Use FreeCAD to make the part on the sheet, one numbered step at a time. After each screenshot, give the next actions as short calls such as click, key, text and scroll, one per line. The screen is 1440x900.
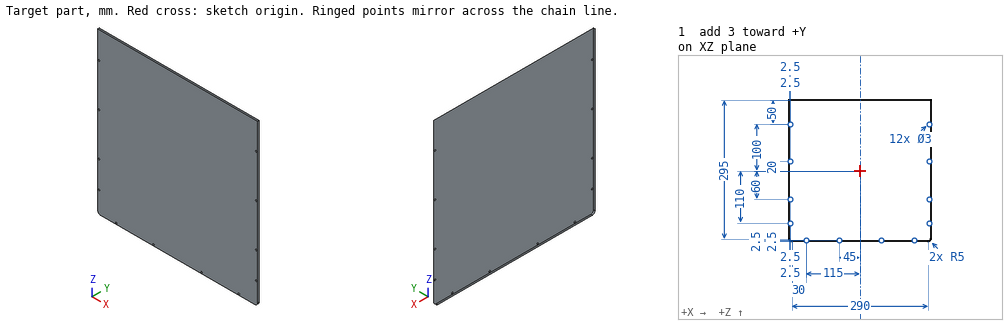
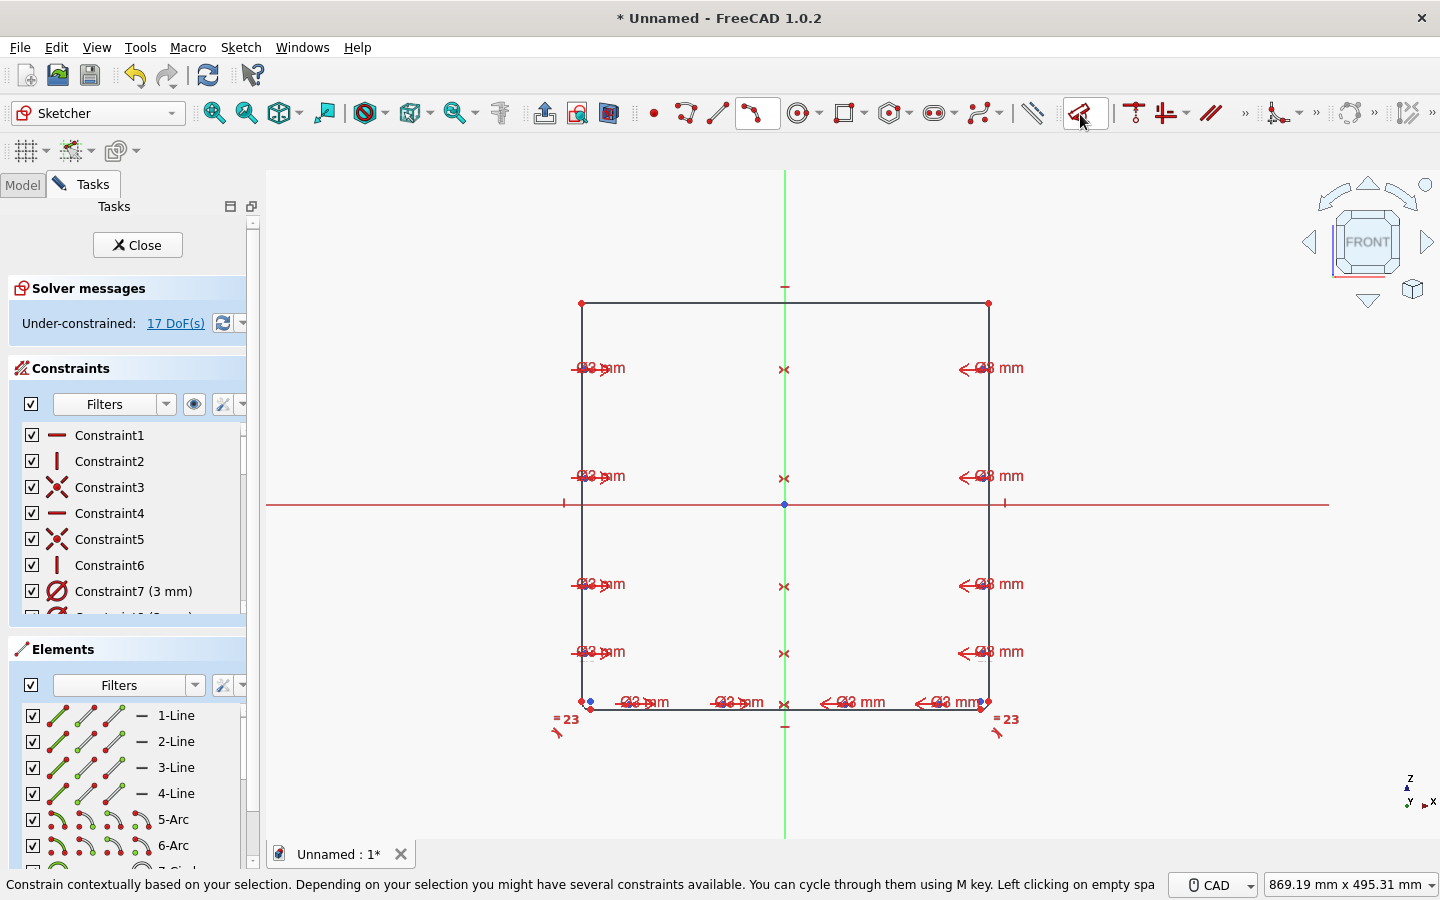
scroll(584, 708, up, 9)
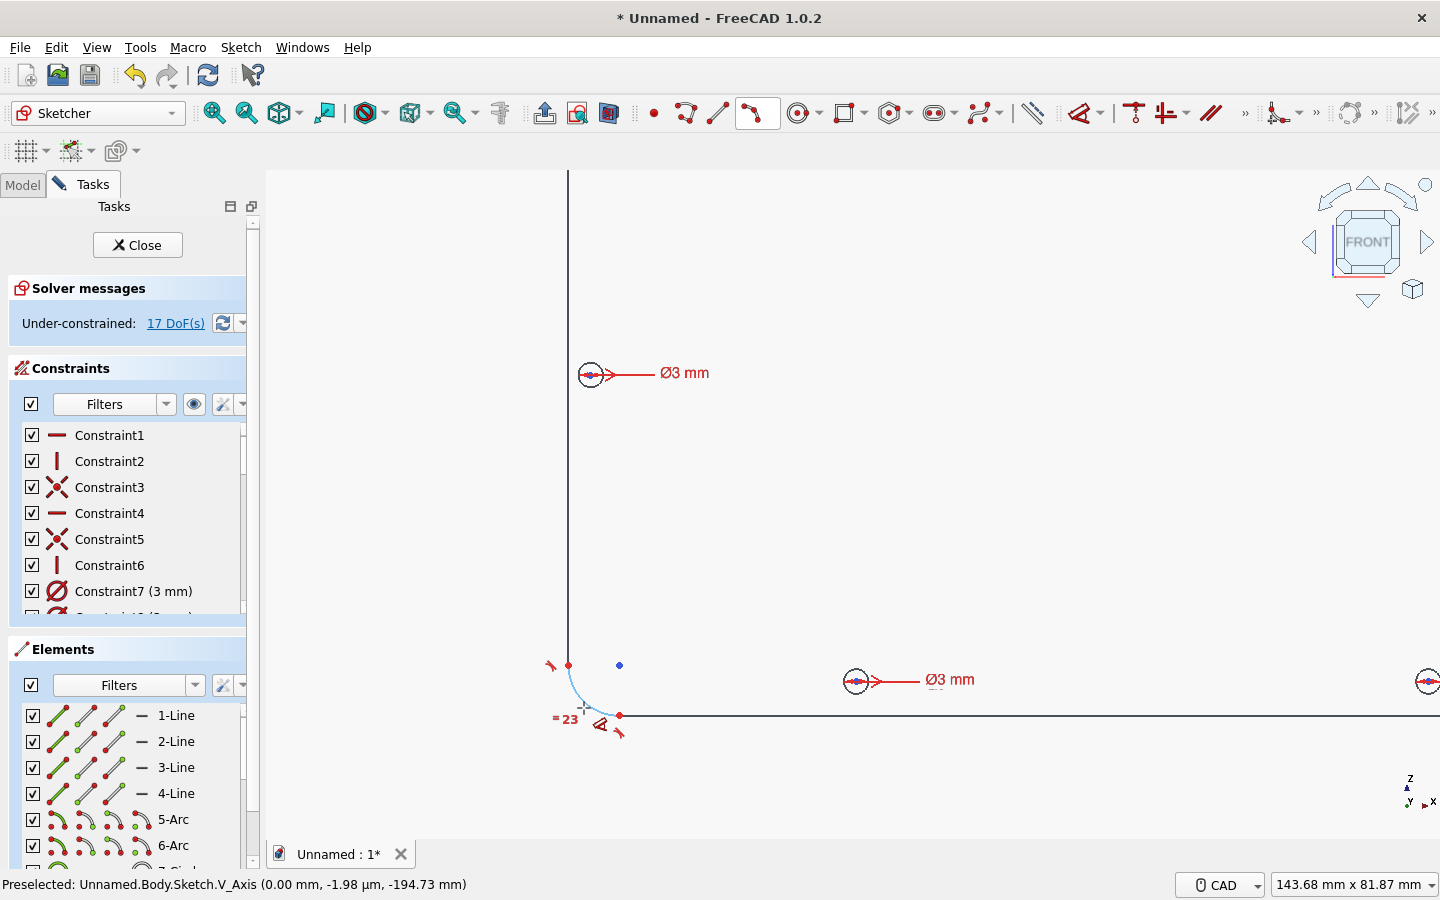
click(583, 701)
click(560, 724)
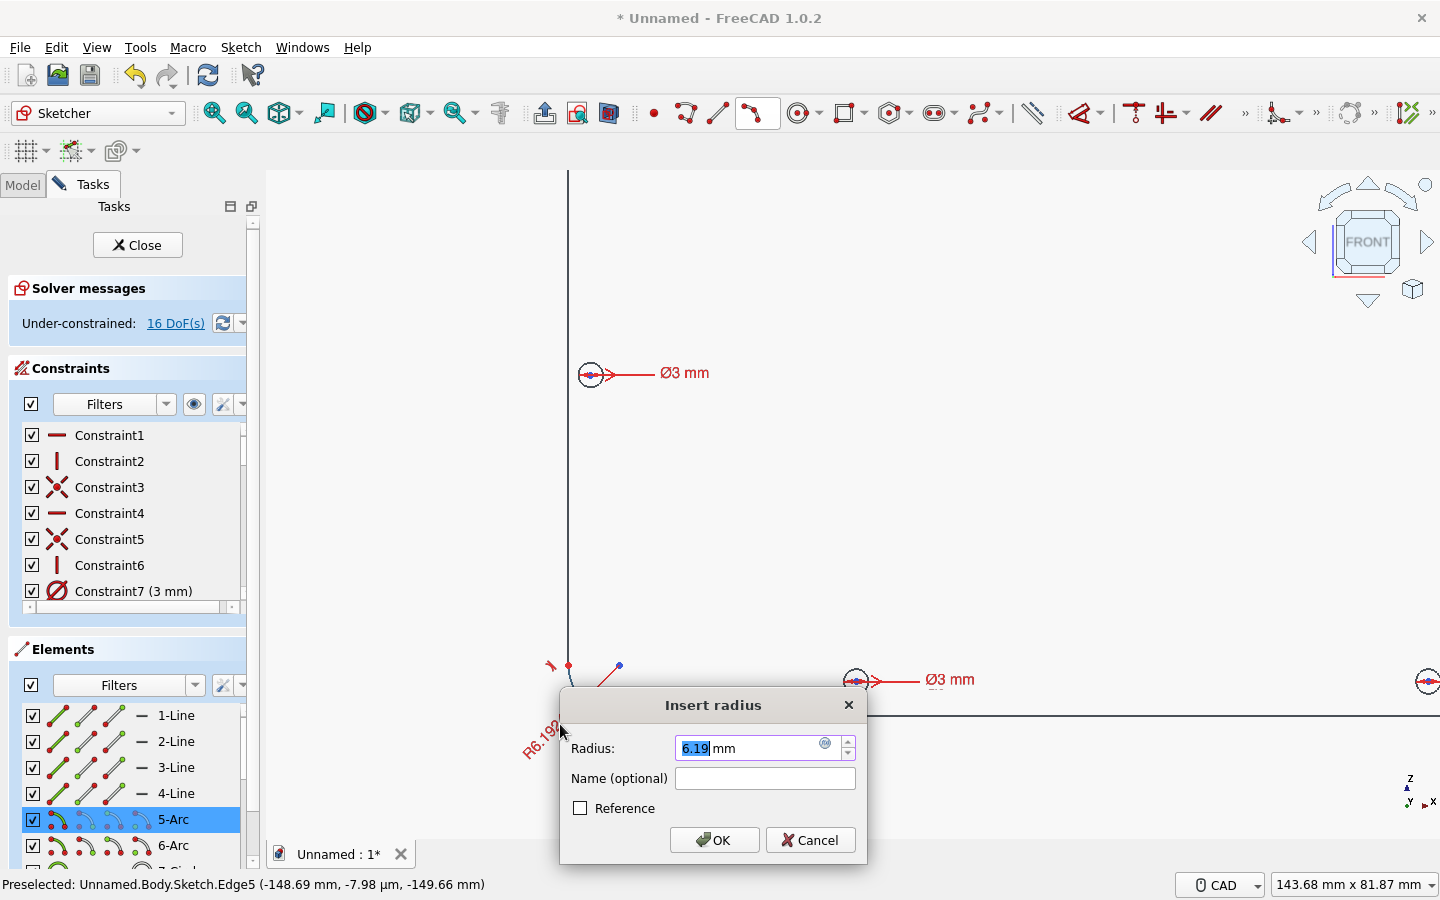
text(5)
key(Return)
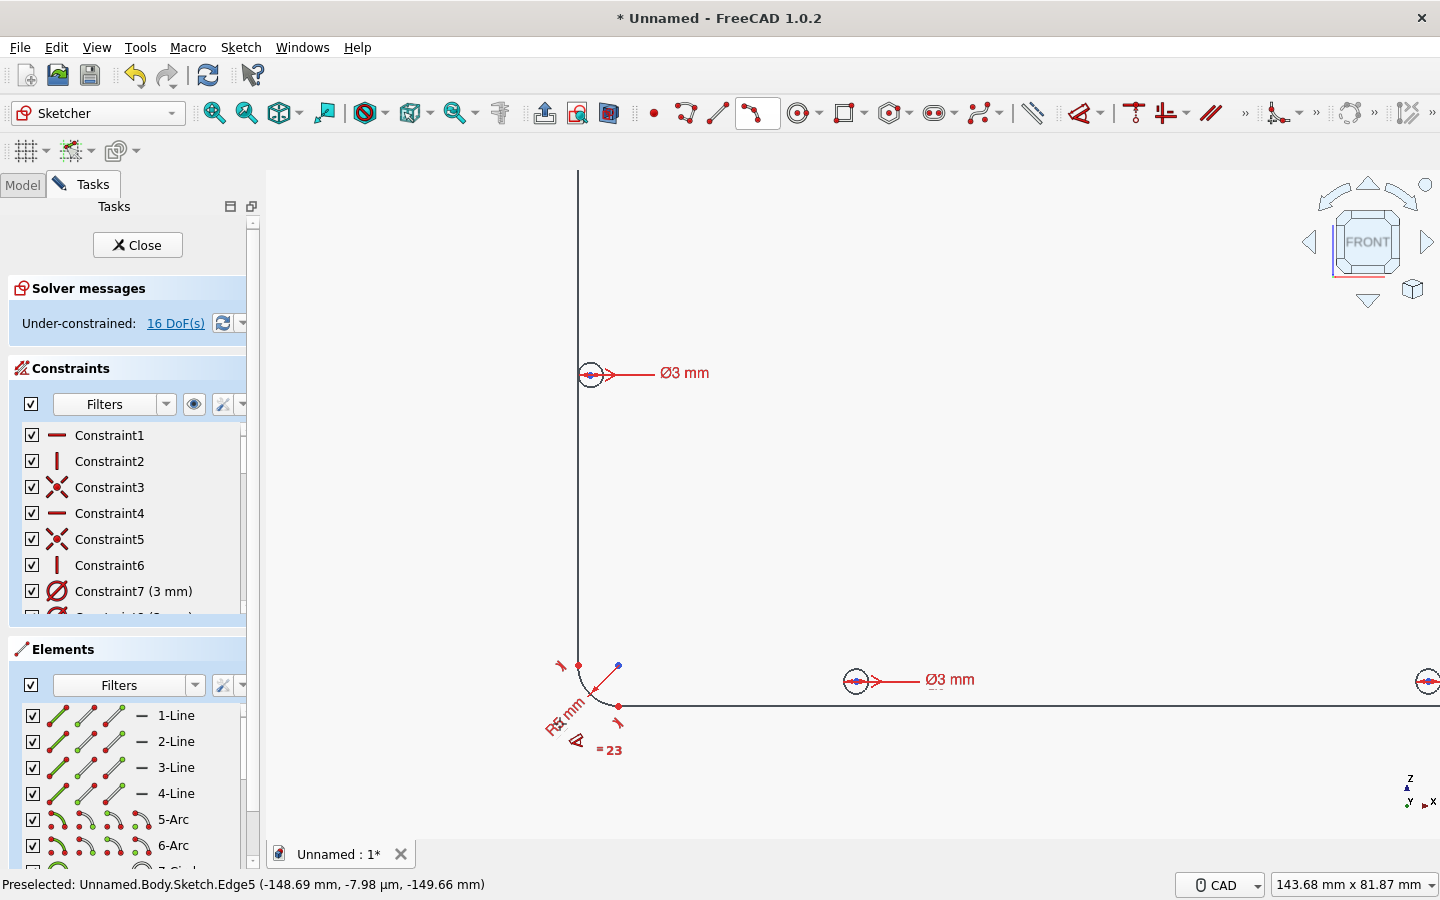
scroll(584, 708, down, 9)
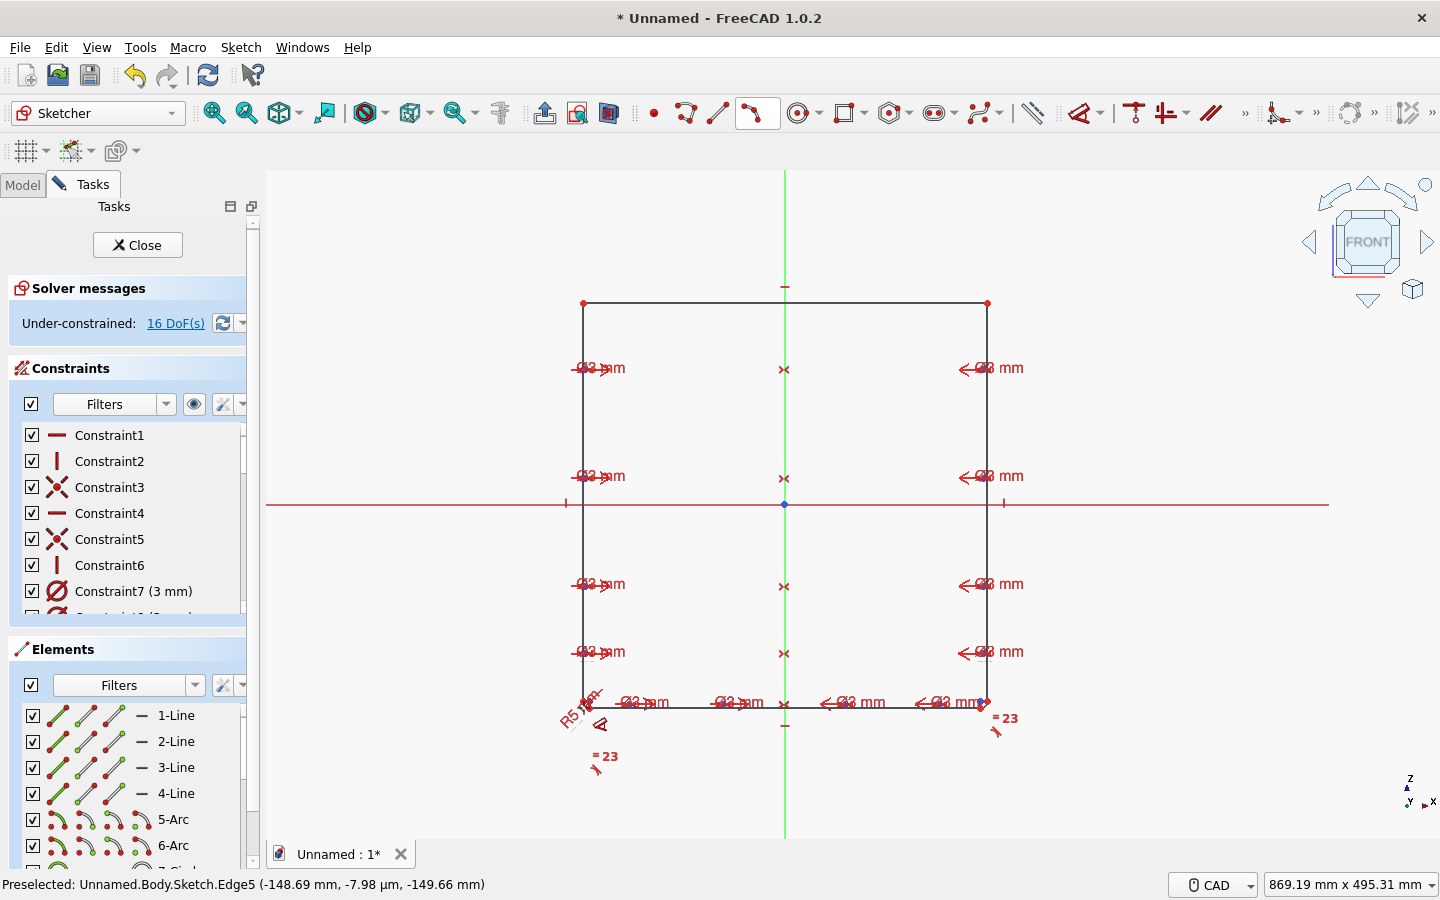
scroll(585, 478, up, 2)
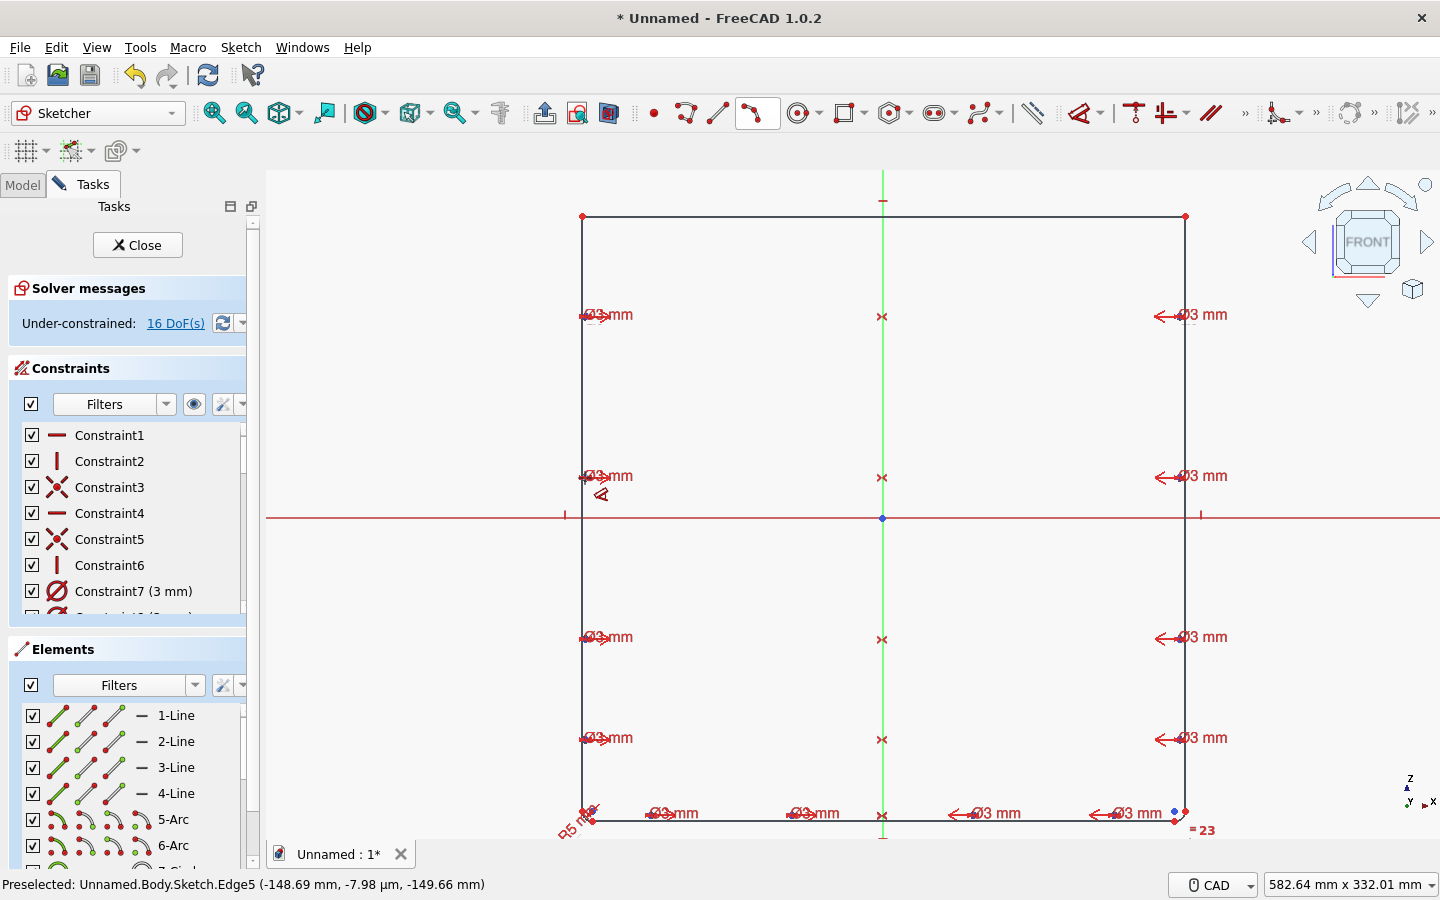
click(585, 478)
click(551, 498)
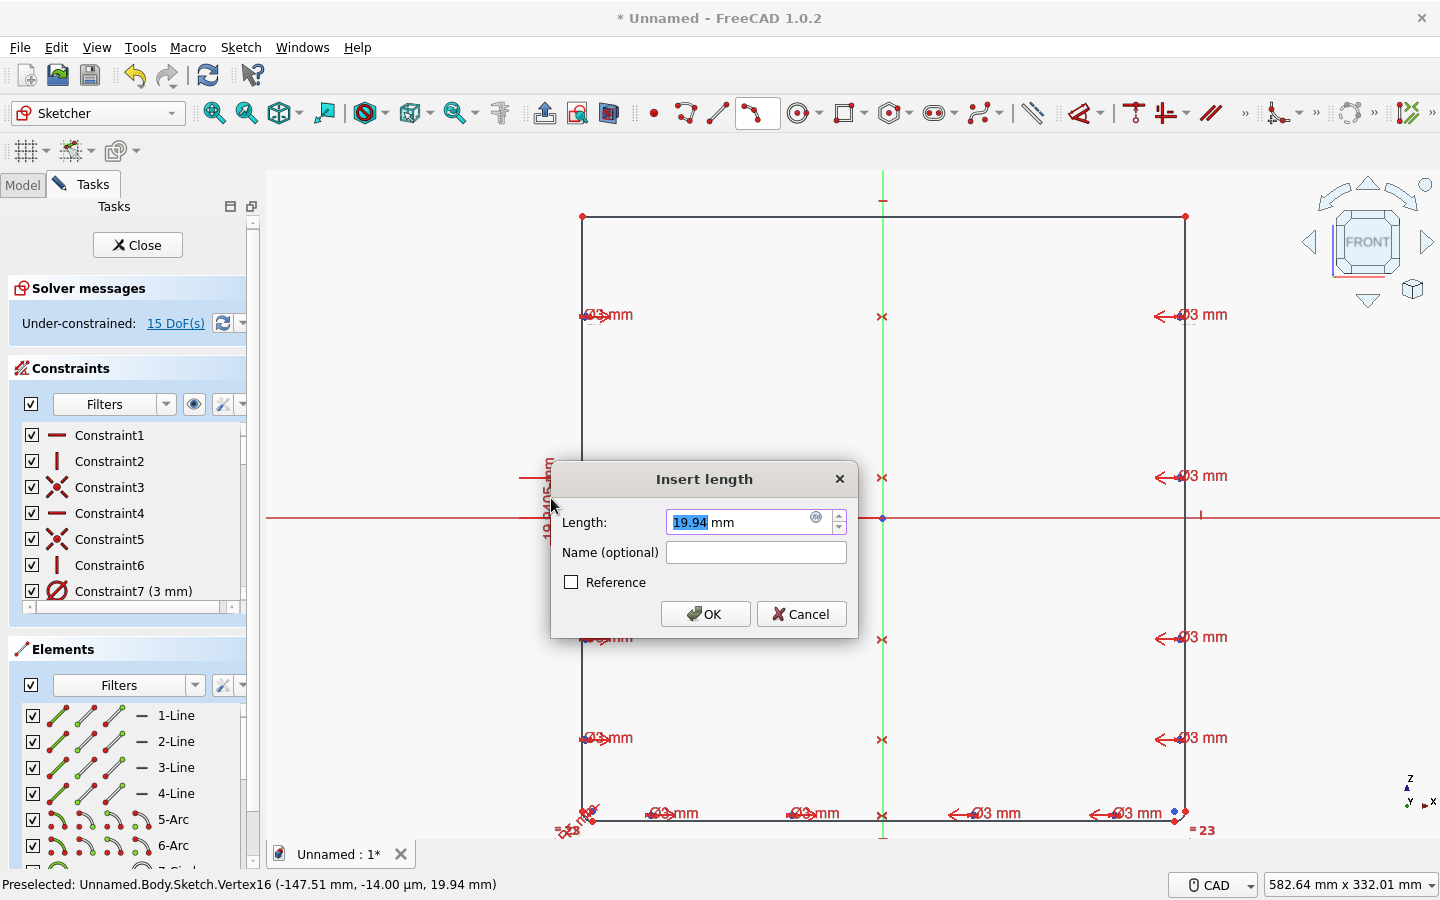
text(20)
key(Return)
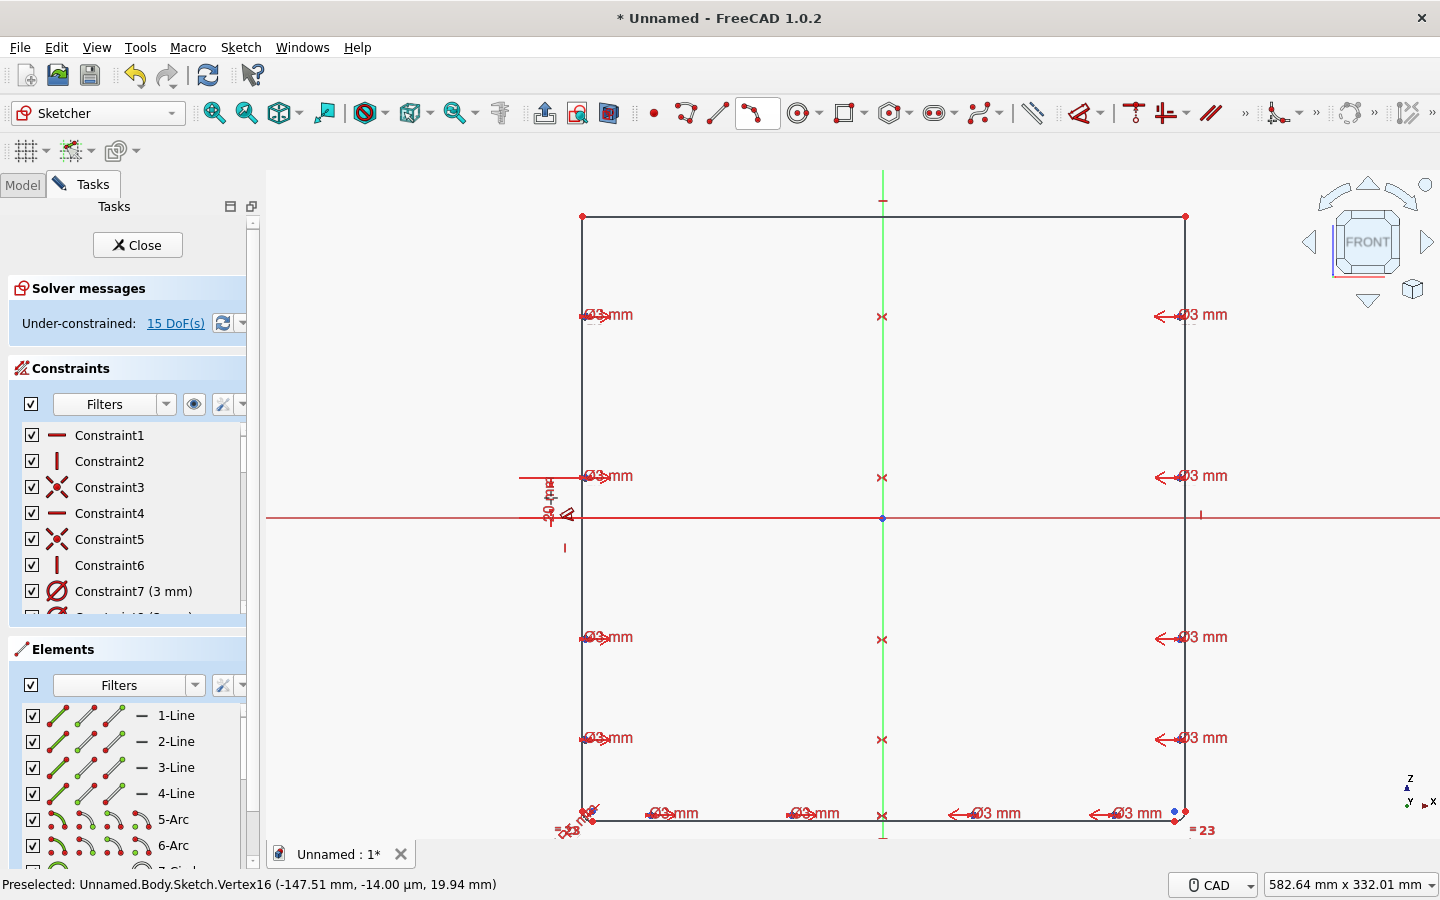
click(585, 639)
click(551, 579)